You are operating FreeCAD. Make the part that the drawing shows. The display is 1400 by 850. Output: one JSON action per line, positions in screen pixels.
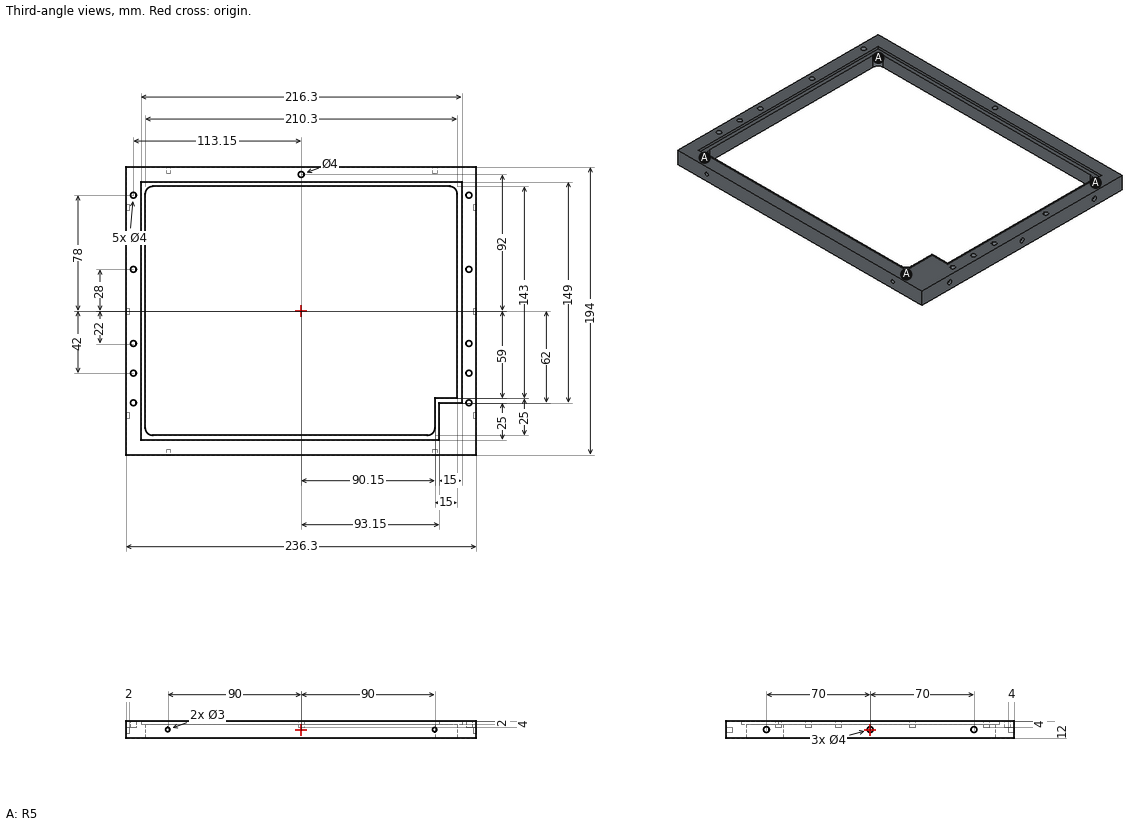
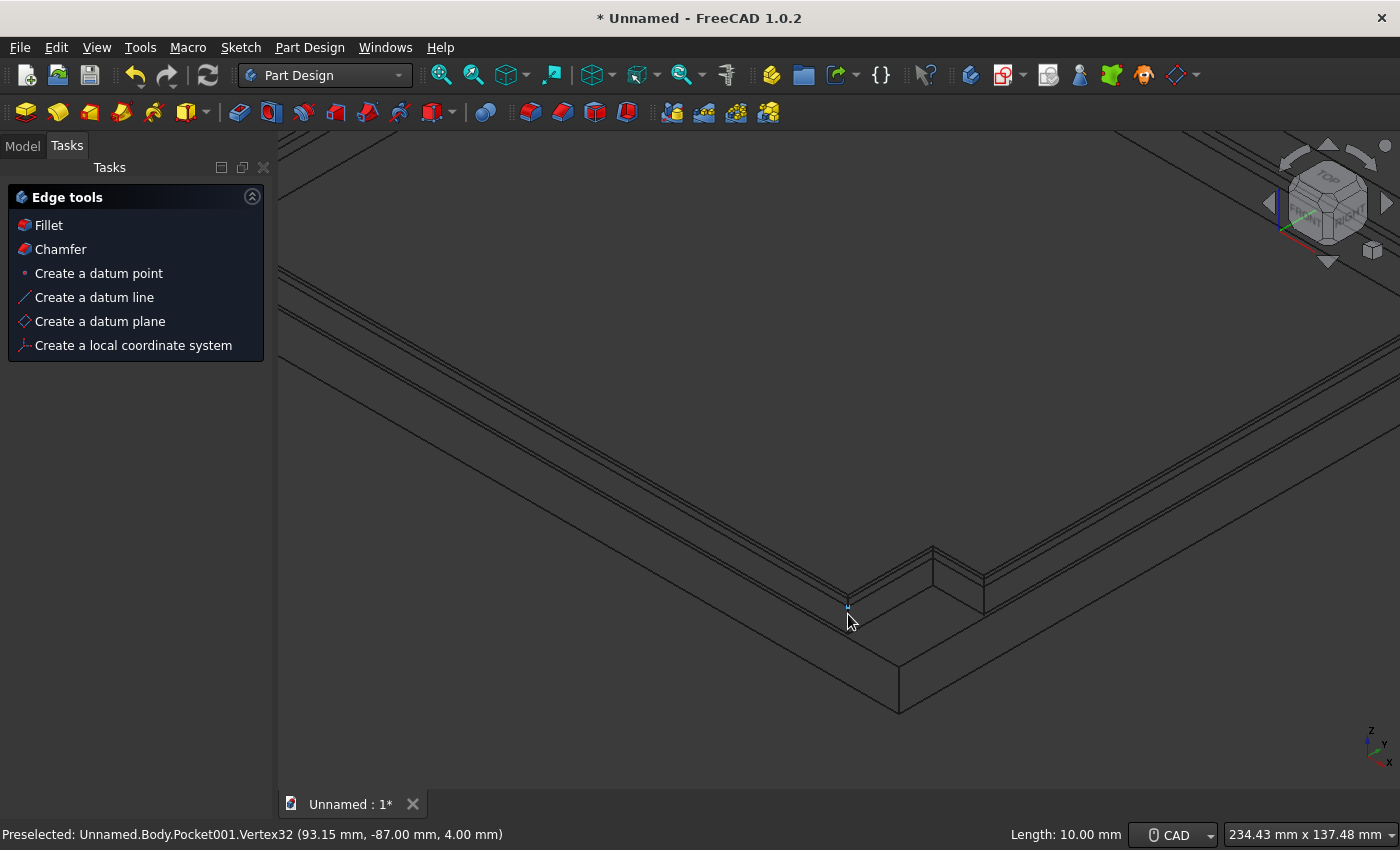
{"action": "left_click", "coordinate": [848, 614], "text": "ctrl"}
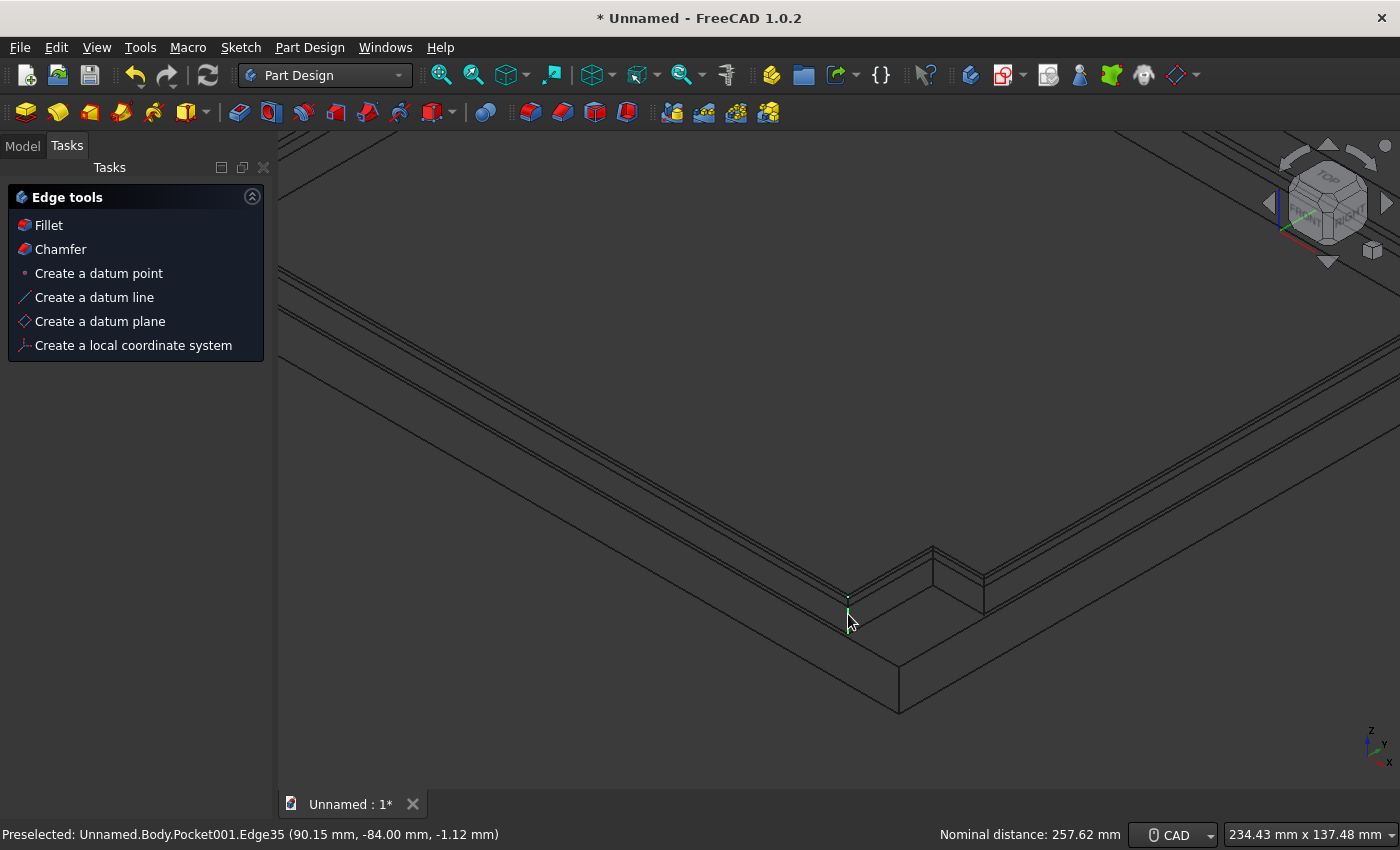
{"action": "left_click", "coordinate": [442, 76]}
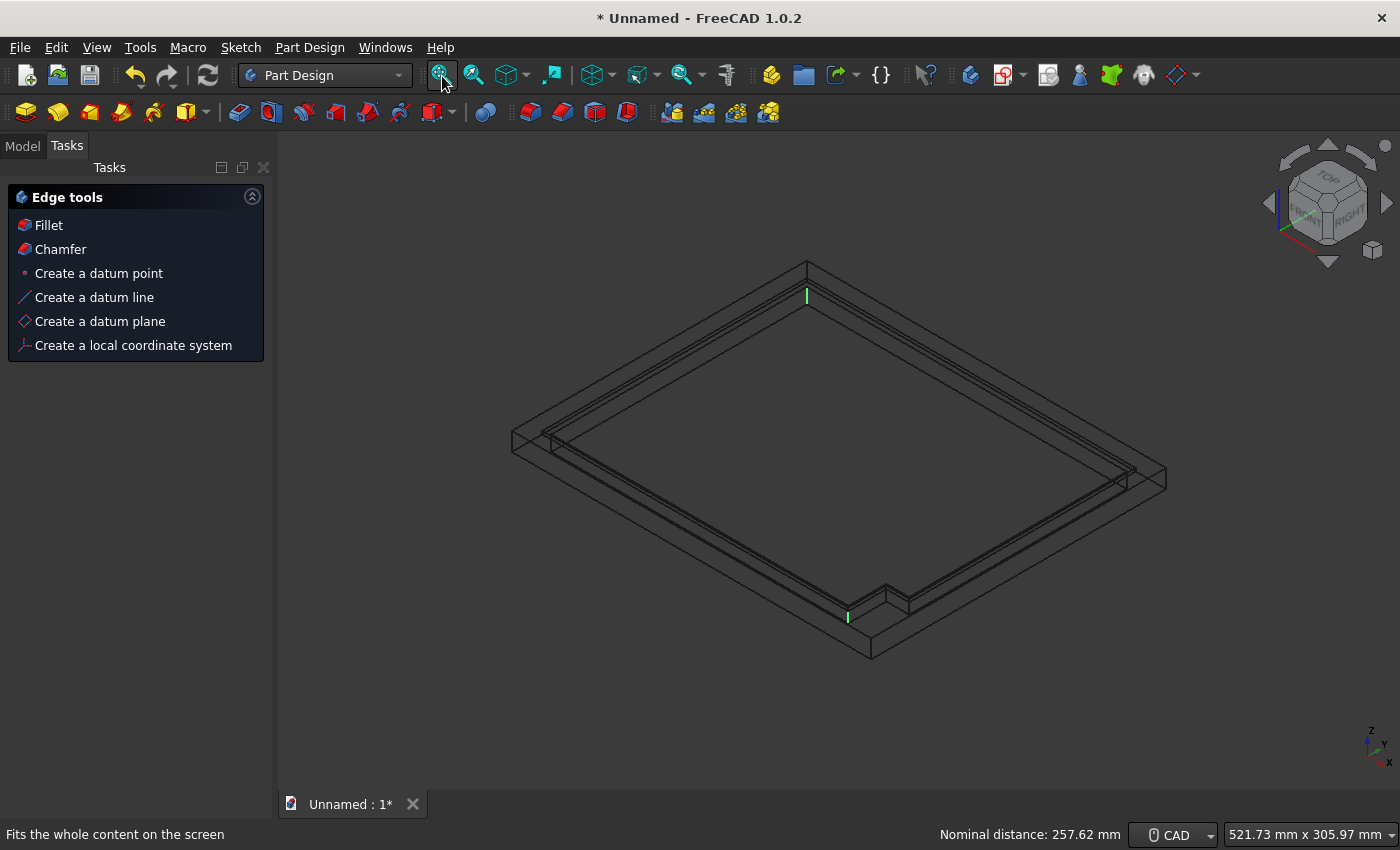
{"action": "key", "text": "2"}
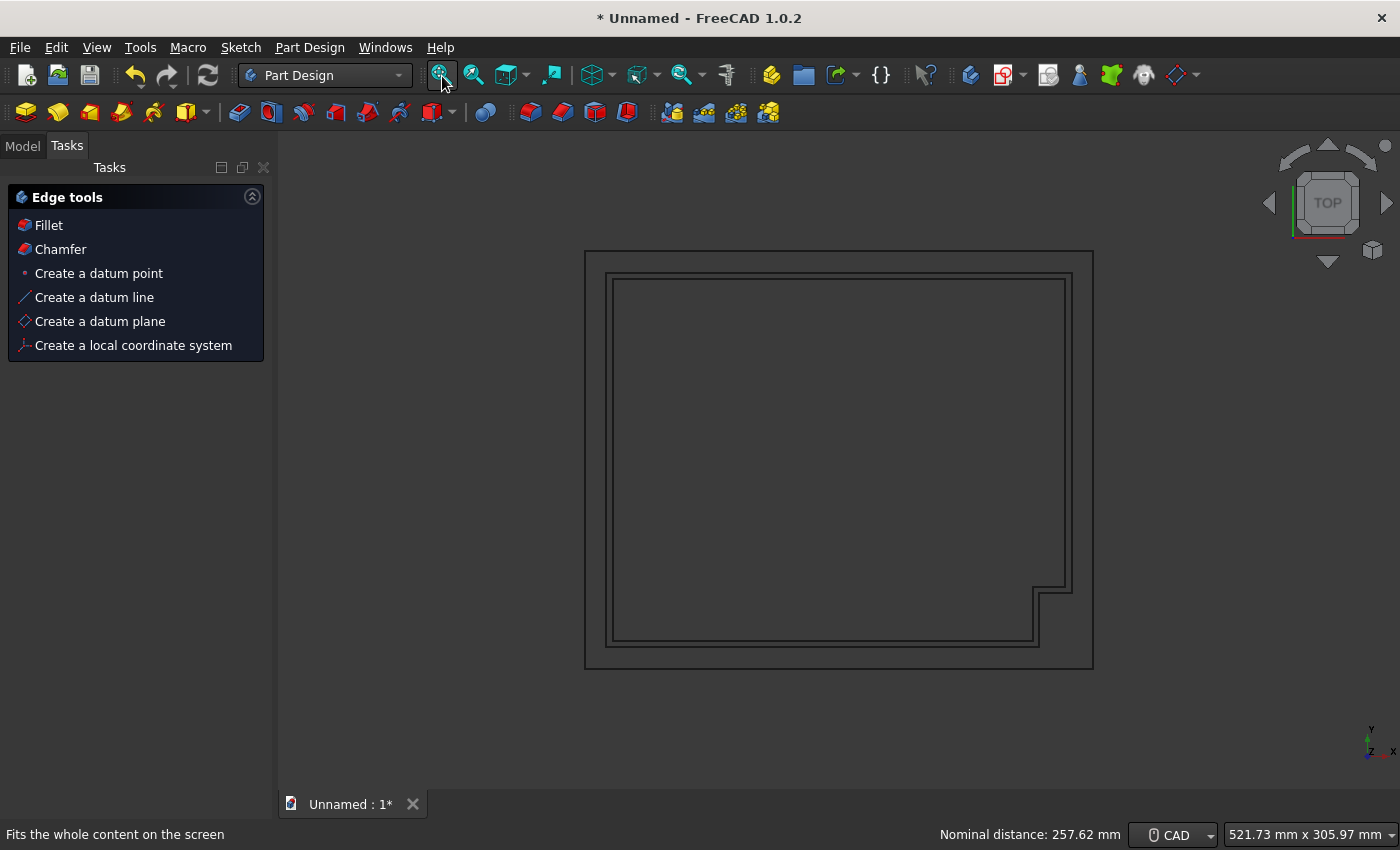
{"action": "scroll", "coordinate": [613, 640], "scroll_direction": "up", "scroll_amount": 4}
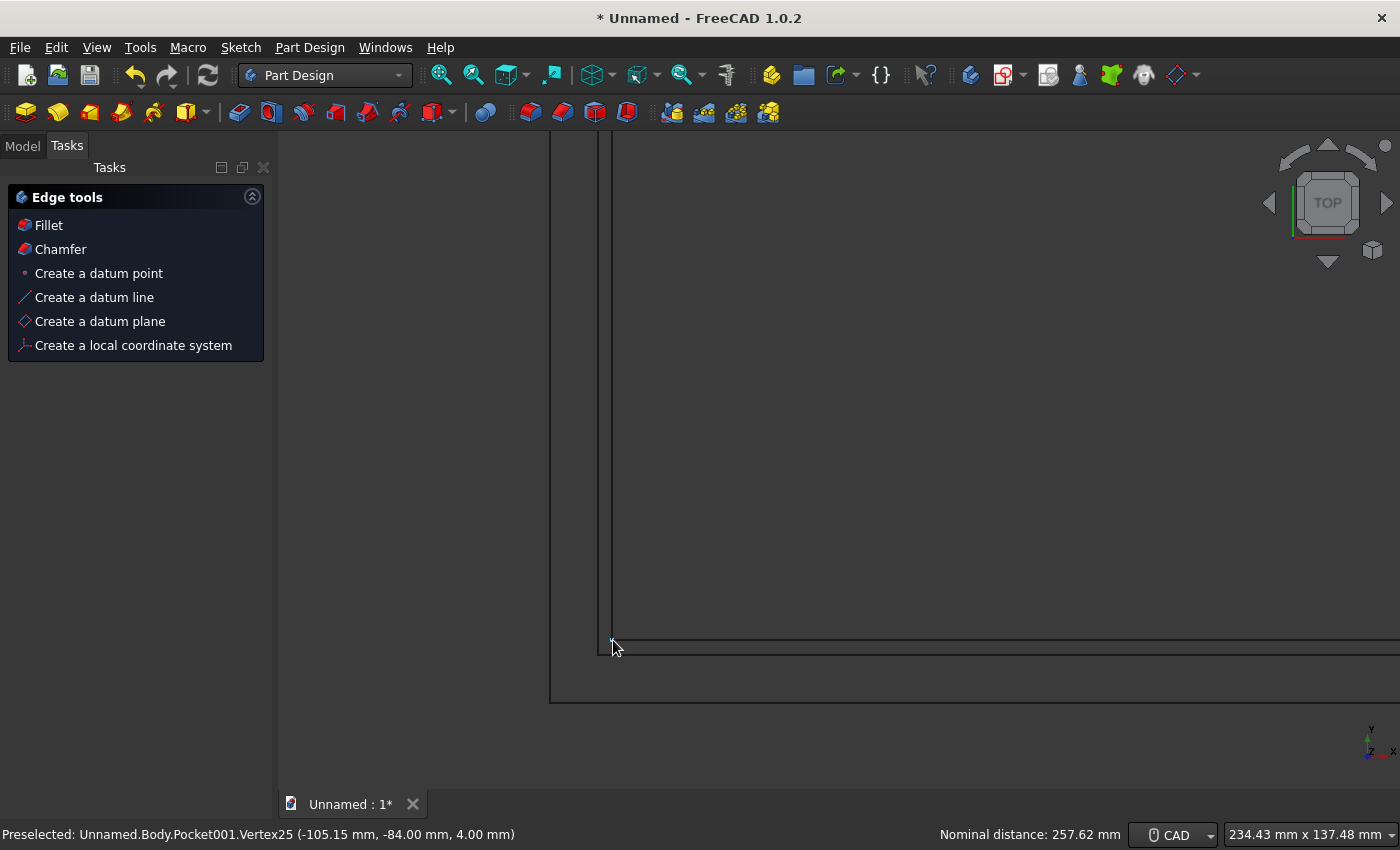
{"action": "left_click", "coordinate": [442, 76]}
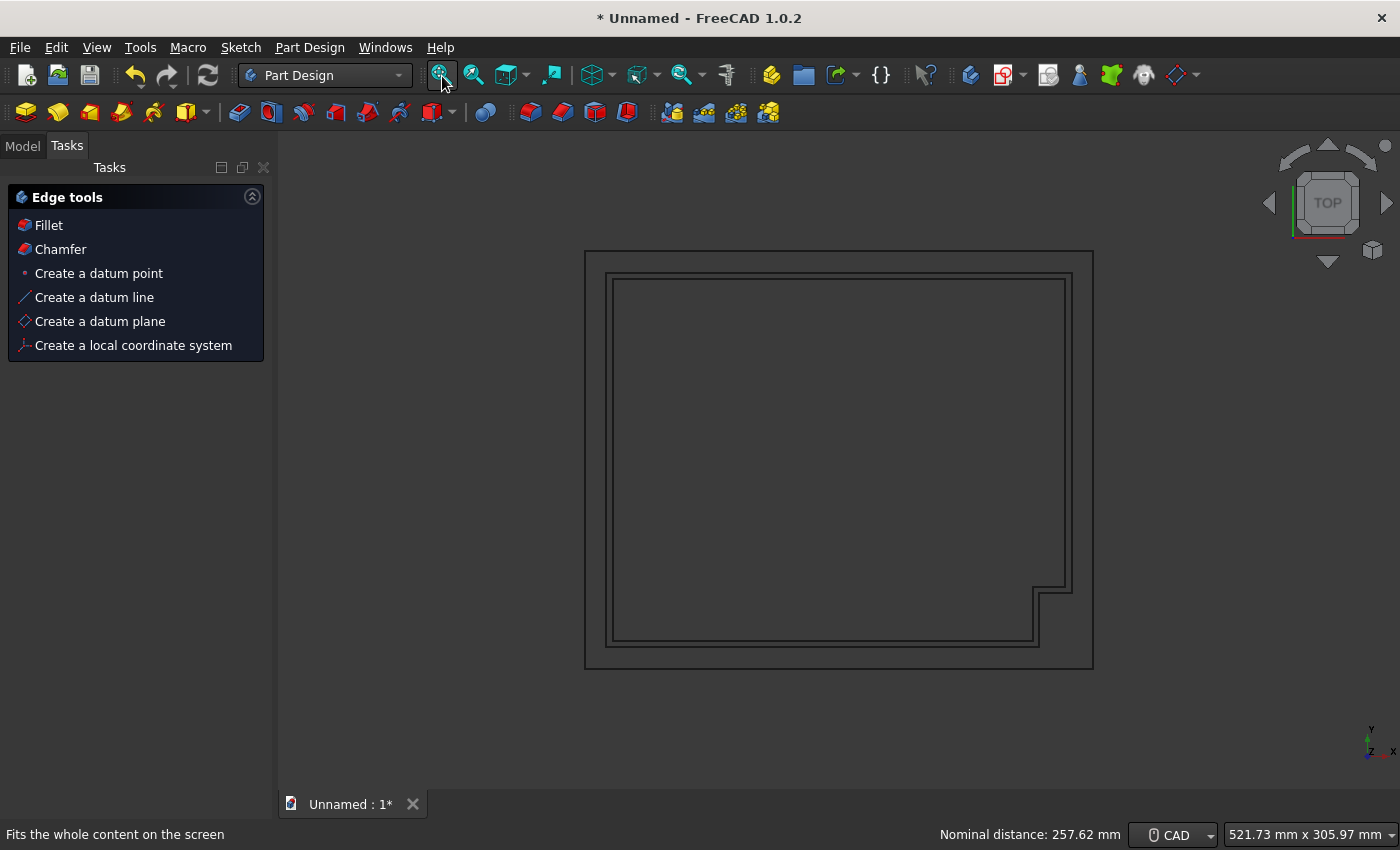
{"action": "key", "text": "1"}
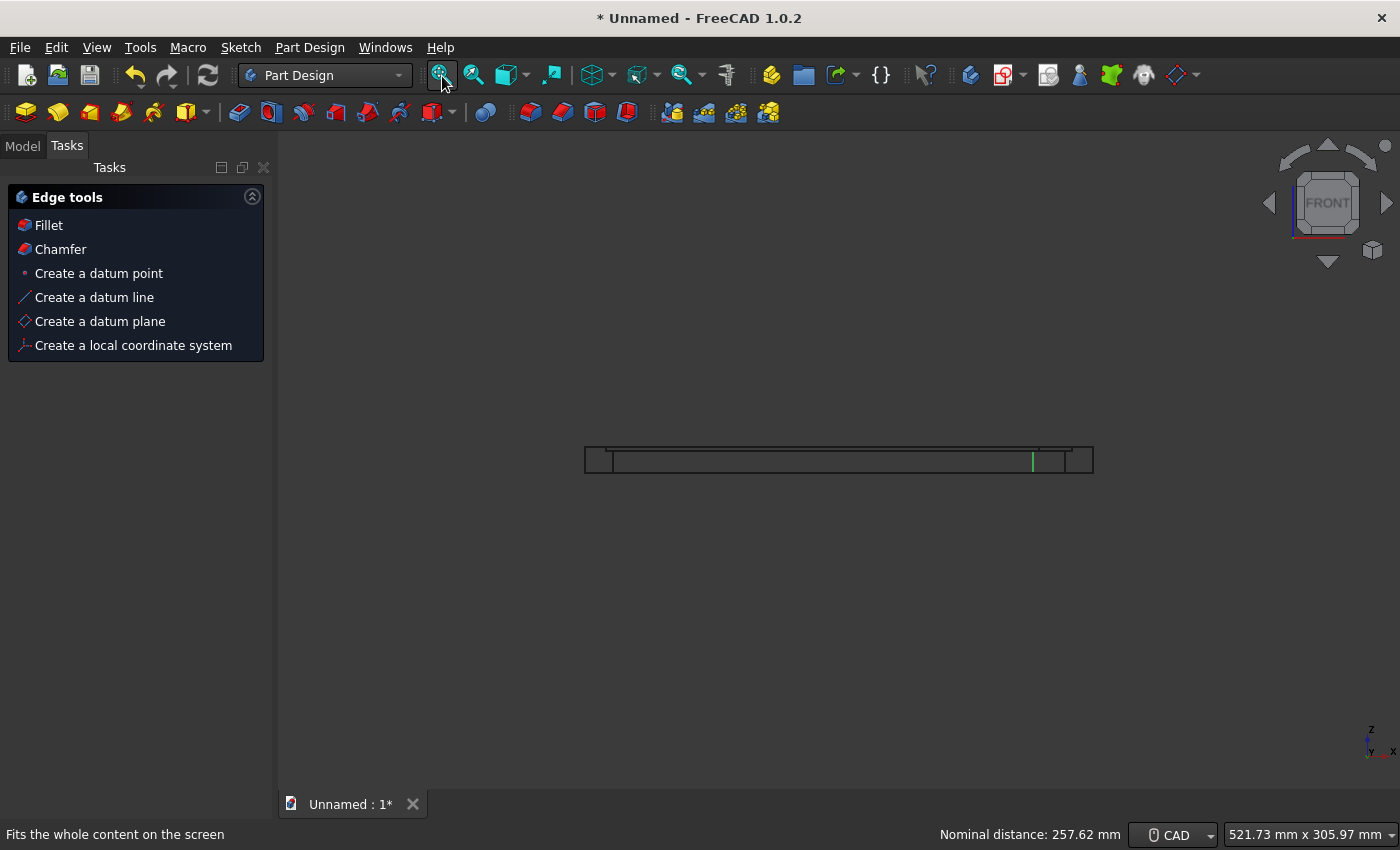
{"action": "left_click", "coordinate": [613, 461], "text": "ctrl"}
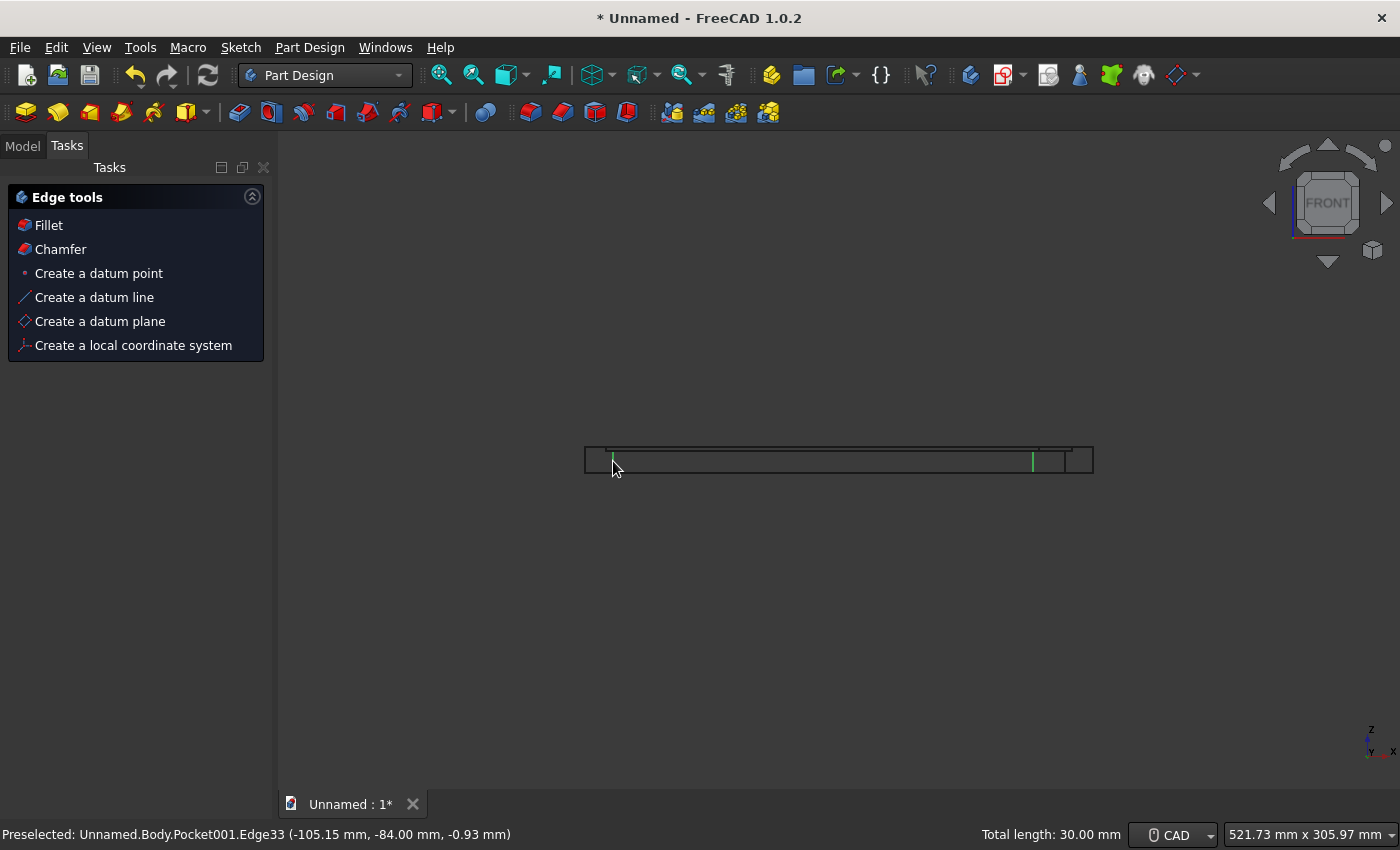
{"action": "scroll", "coordinate": [1065, 461], "scroll_direction": "up", "scroll_amount": 4}